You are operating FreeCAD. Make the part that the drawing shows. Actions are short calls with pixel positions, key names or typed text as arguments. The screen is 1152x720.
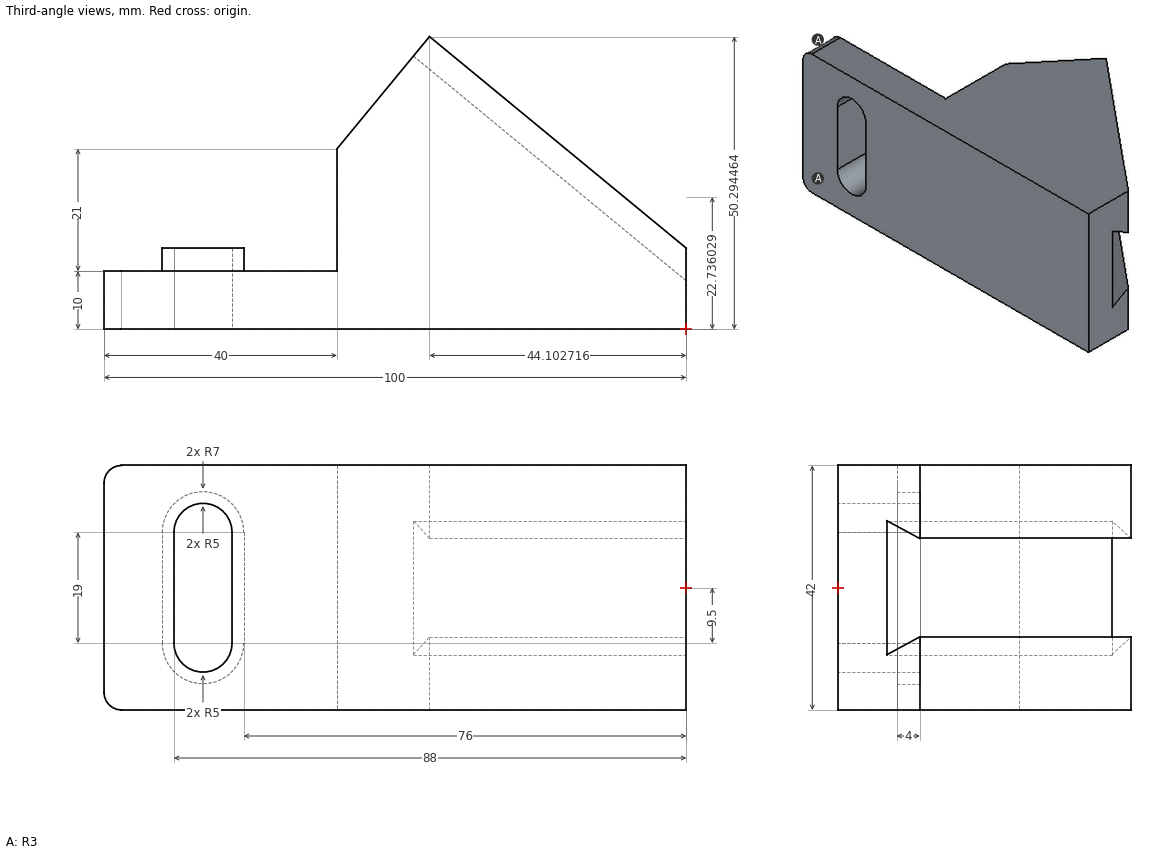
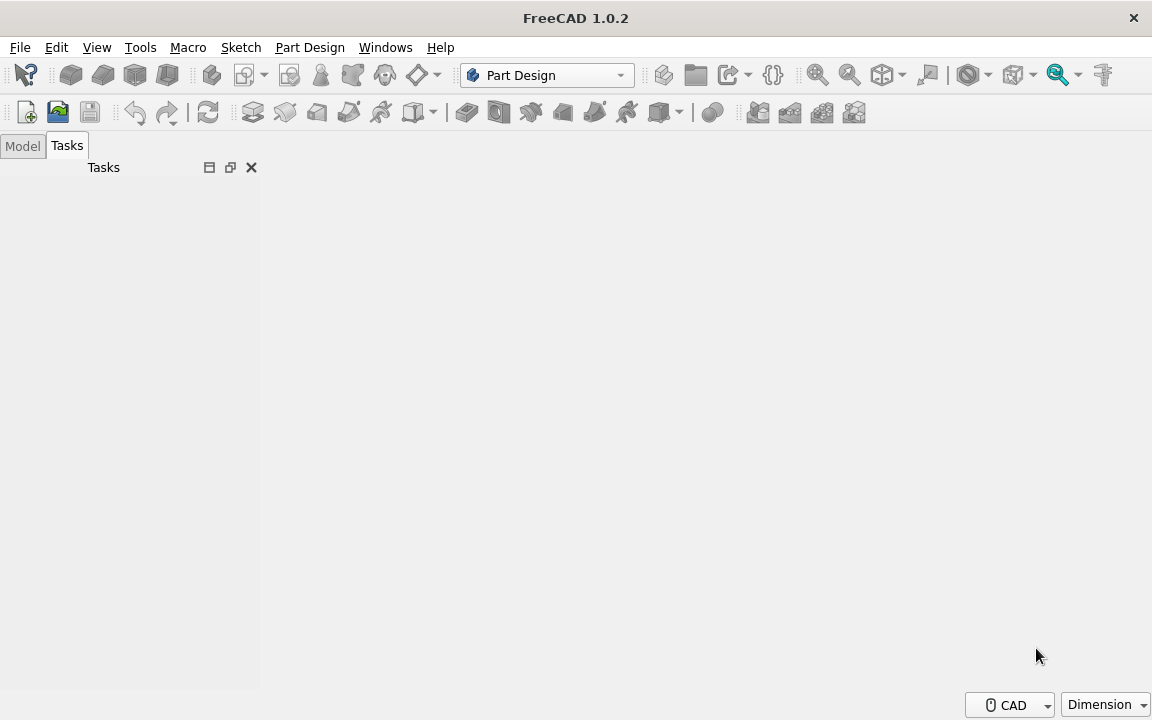
key(ctrl+n)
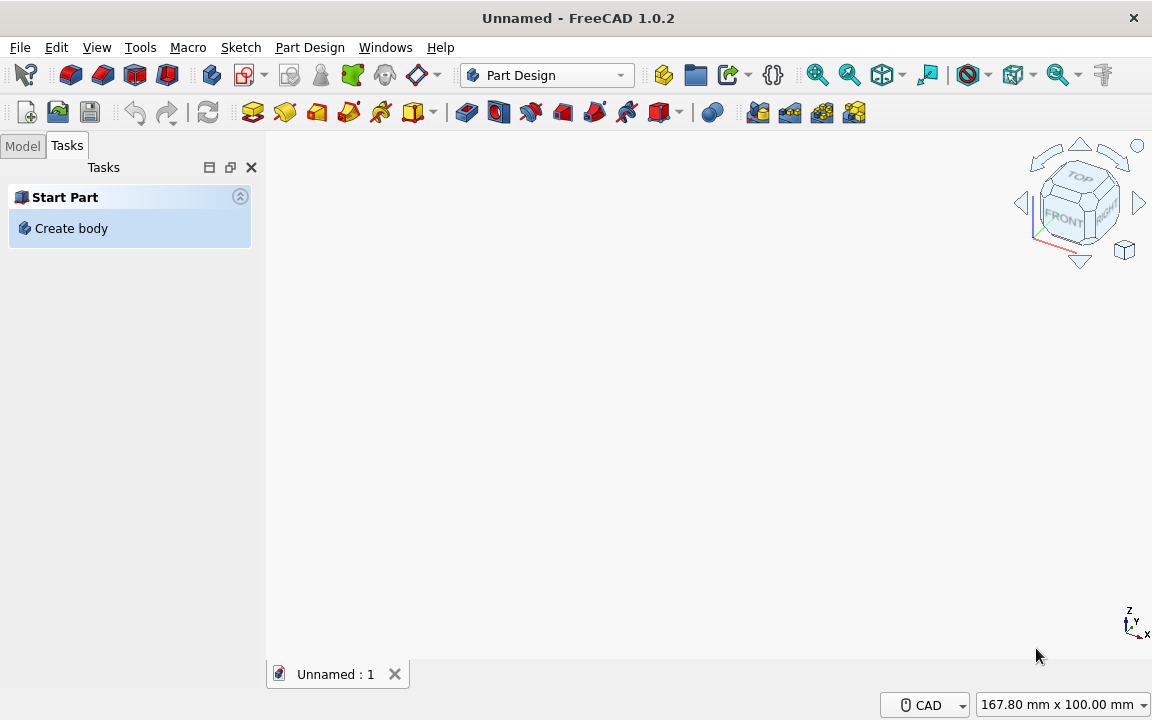
click(244, 76)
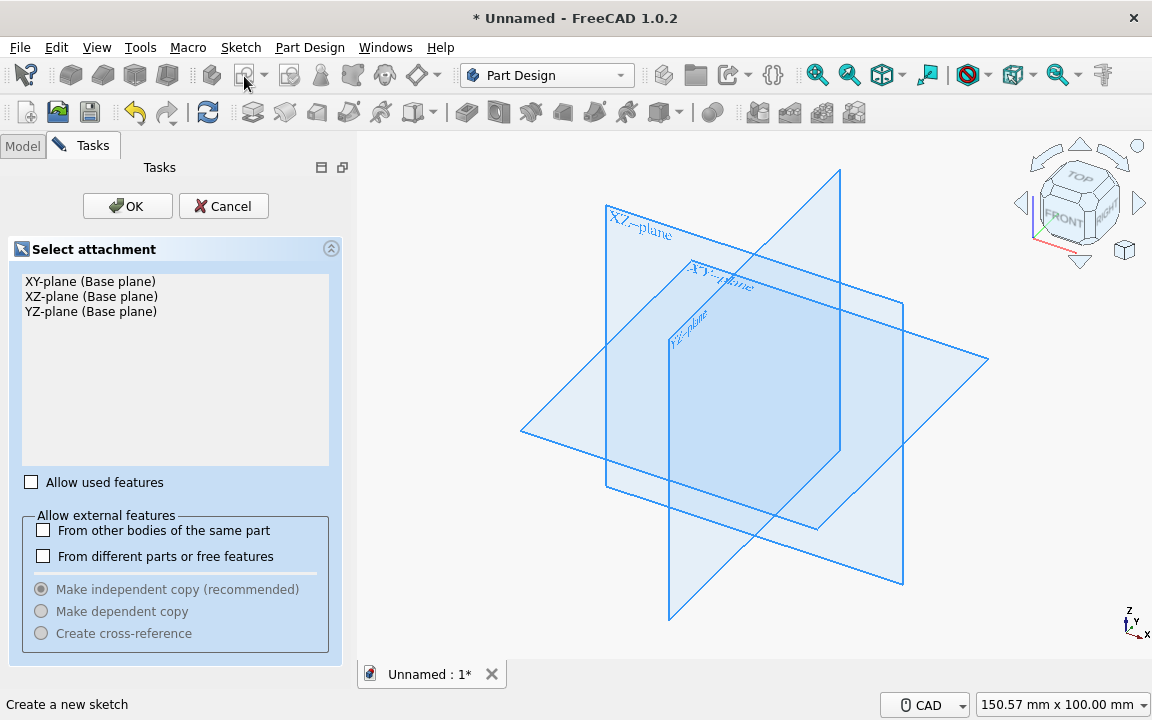
click(82, 282)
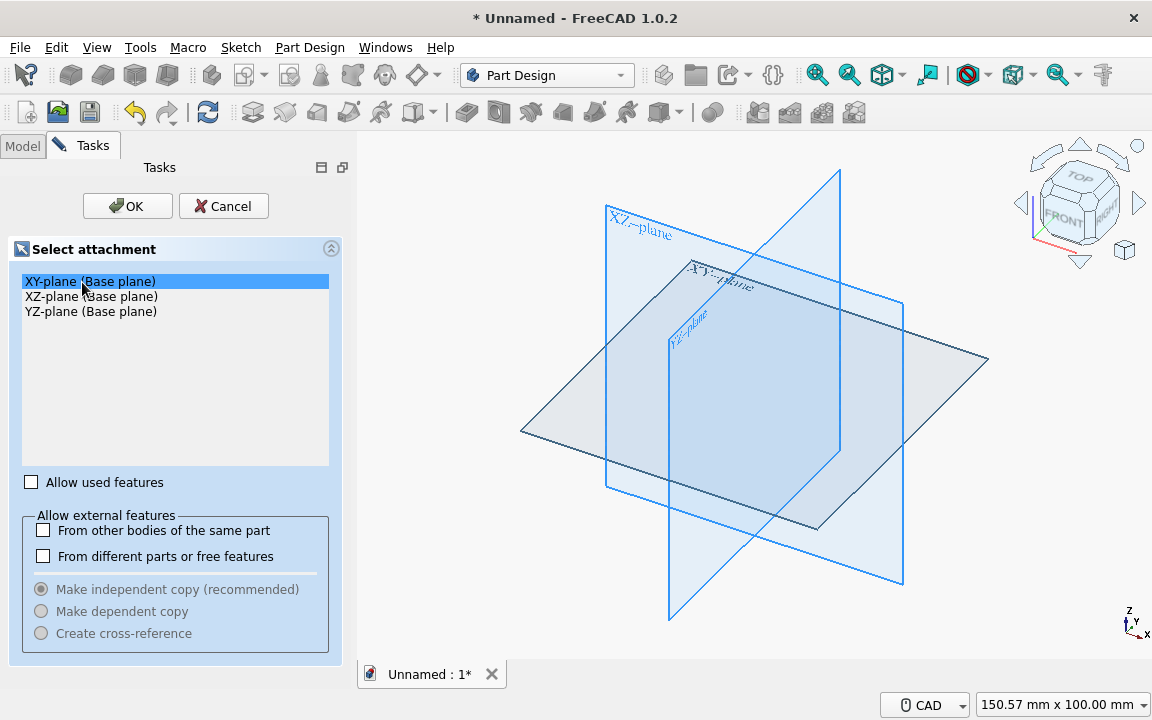
click(128, 206)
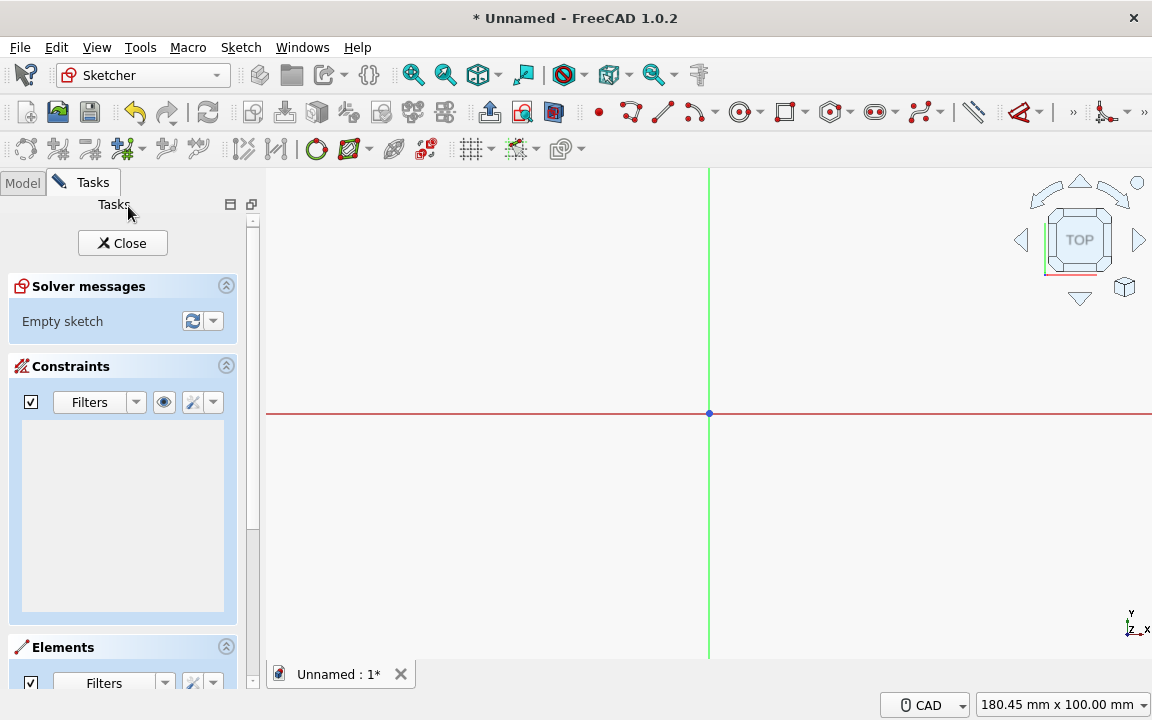
scroll(987, 631, down, 1)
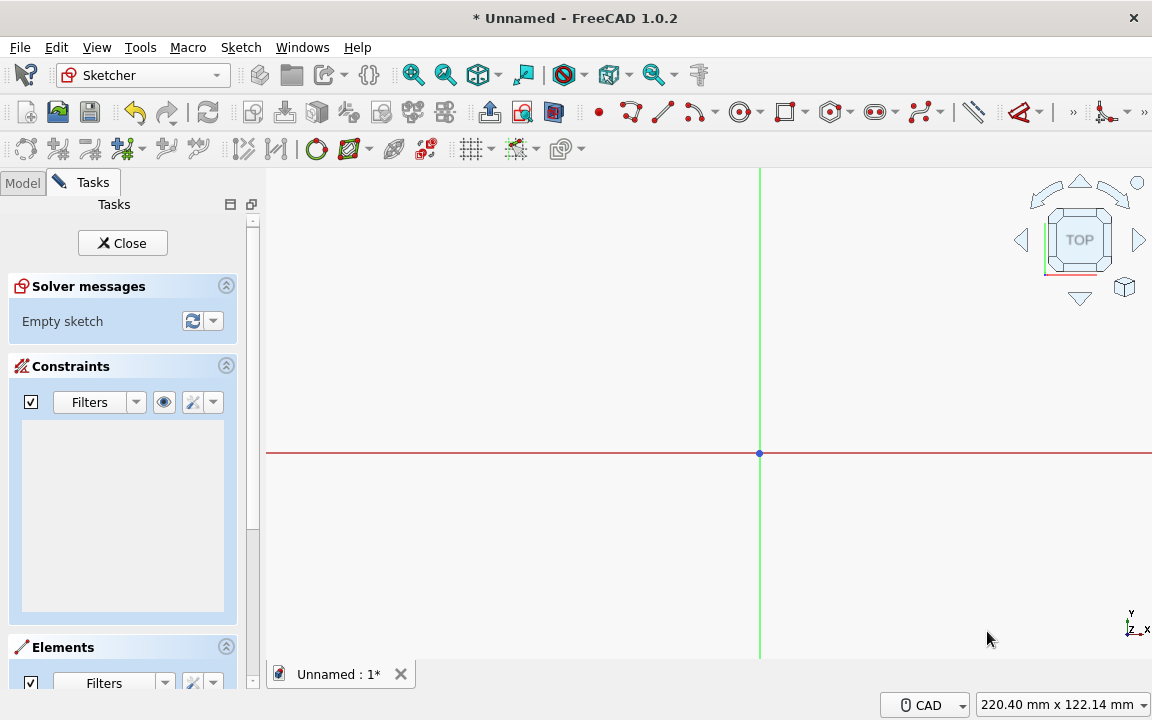
key(g)
key(m)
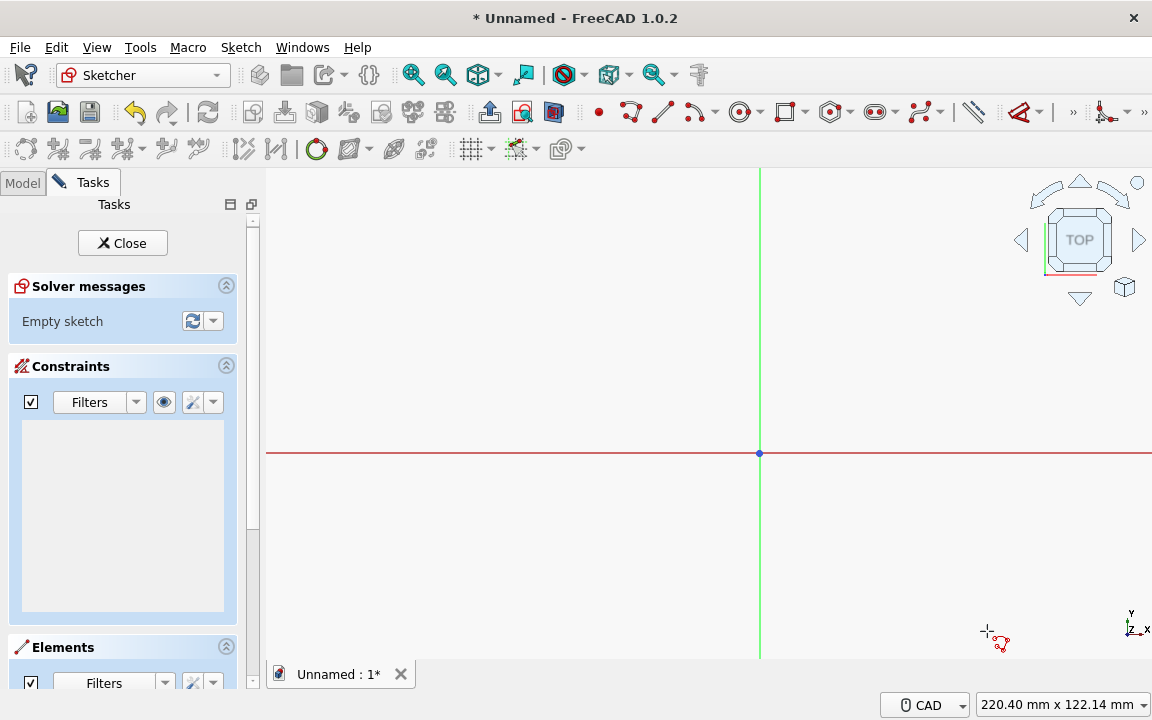
click(760, 453)
click(751, 362)
click(582, 251)
click(518, 328)
click(518, 413)
click(358, 413)
click(358, 444)
click(760, 453)
key(Escape)
key(Escape)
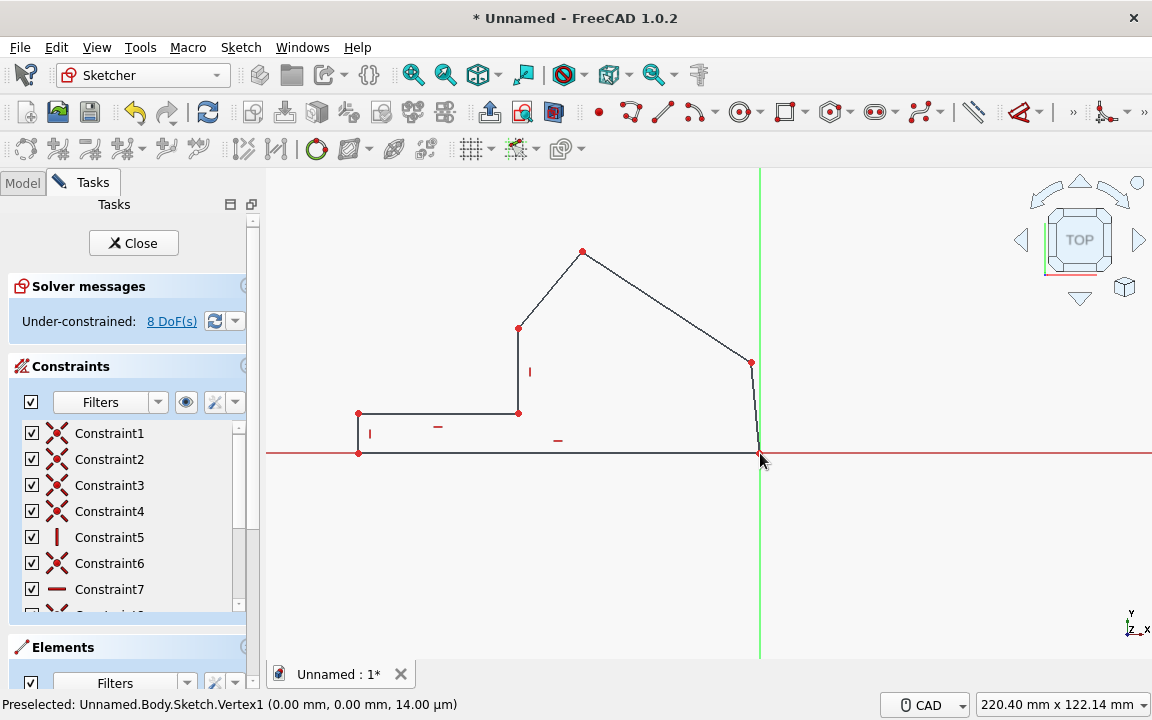
click(757, 426)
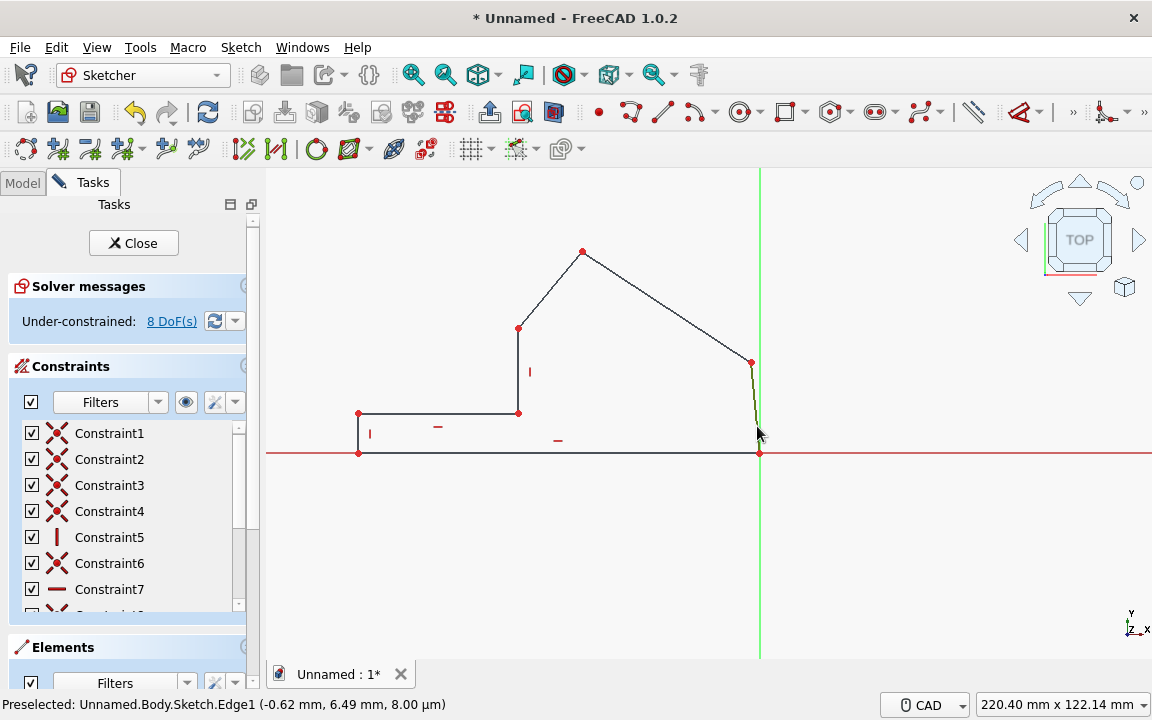
key(v)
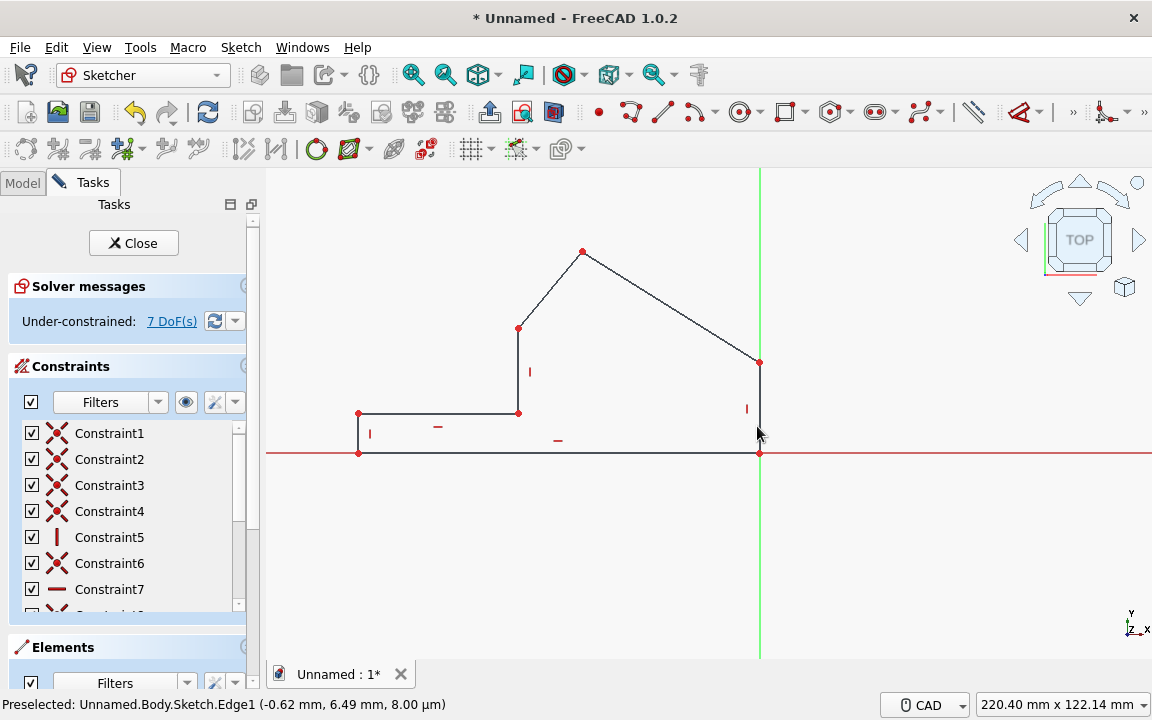
click(1020, 112)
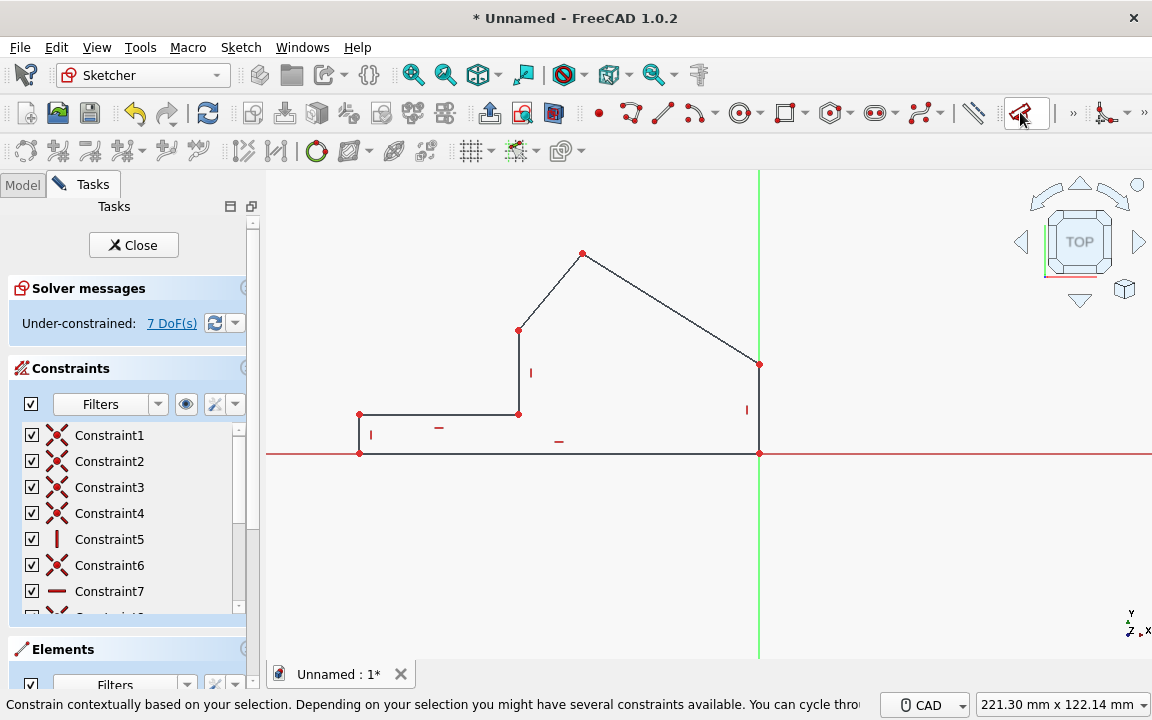
click(519, 356)
click(485, 373)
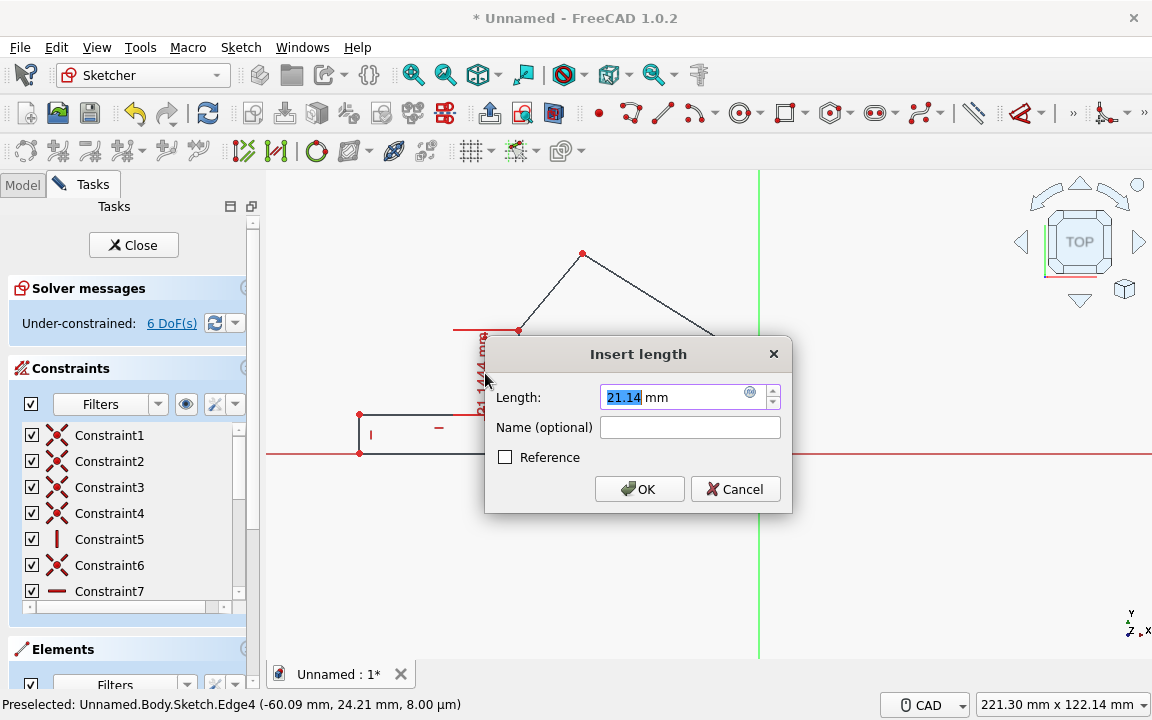
text(21)
key(Return)